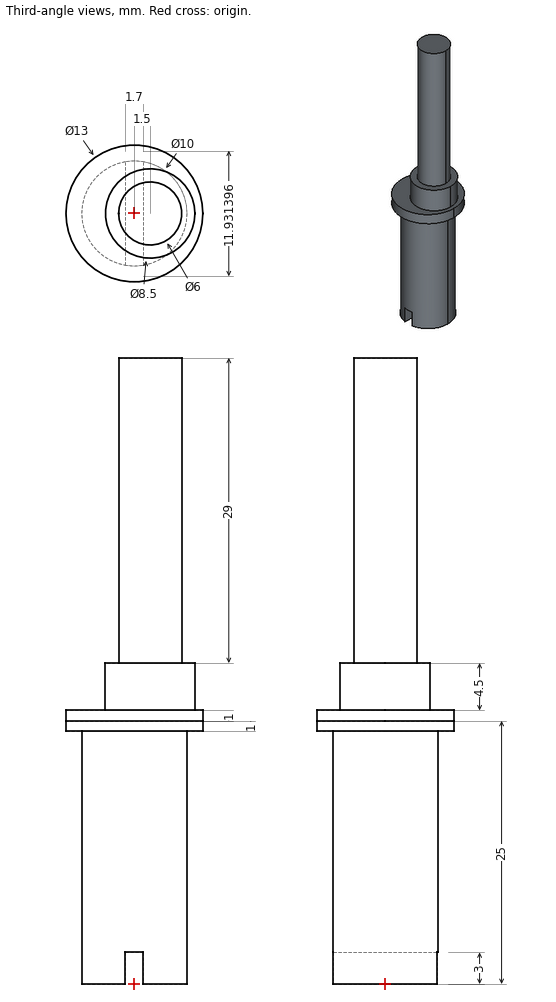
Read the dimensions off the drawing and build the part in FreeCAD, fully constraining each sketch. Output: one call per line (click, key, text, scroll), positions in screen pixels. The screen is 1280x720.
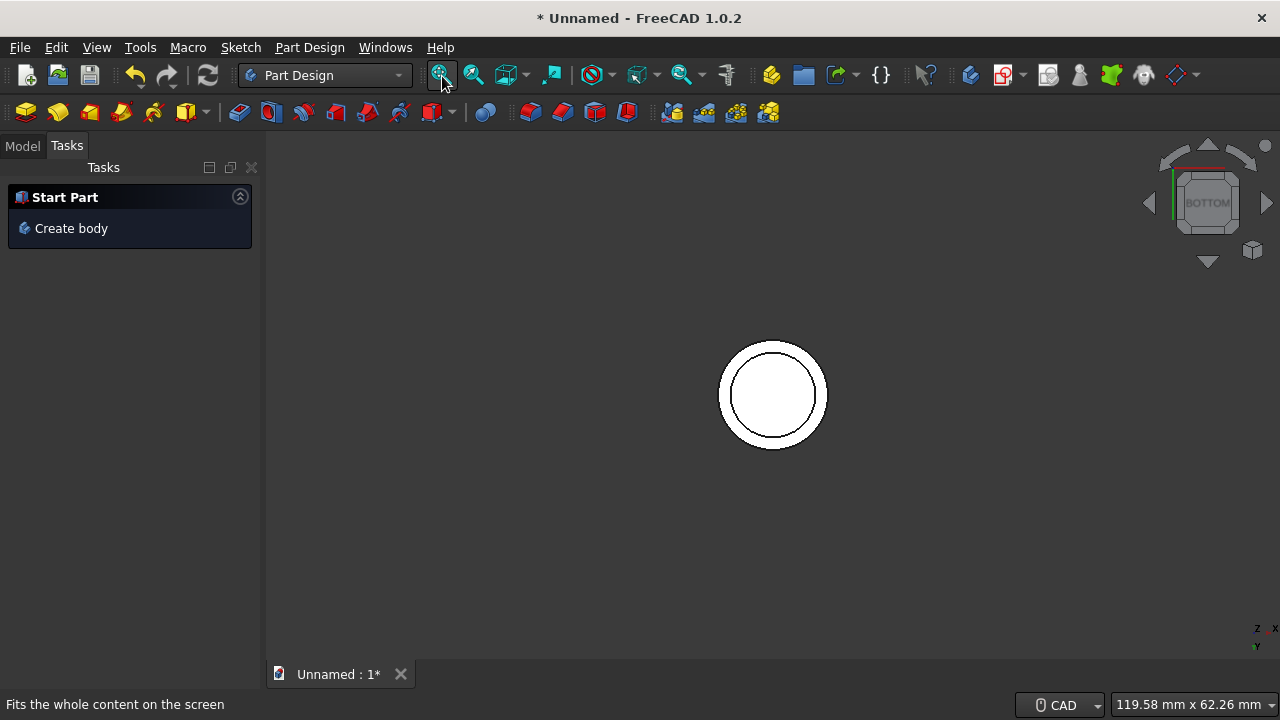
click(442, 76)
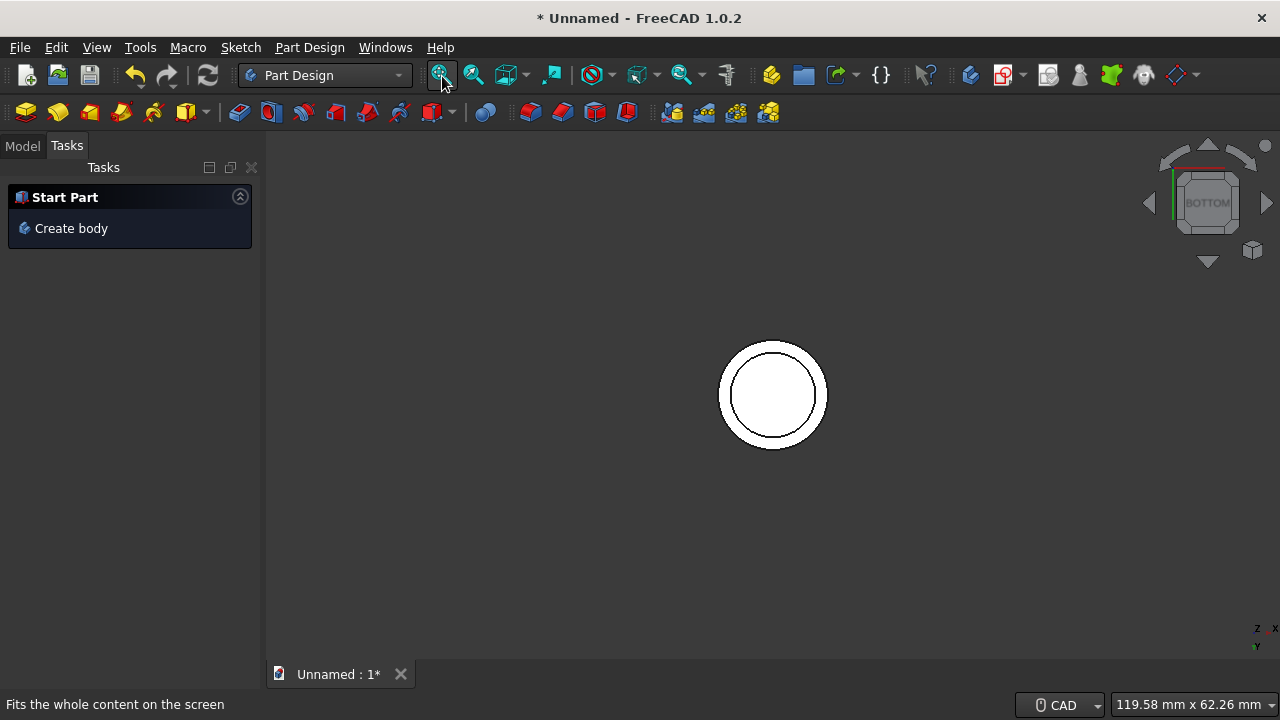
click(773, 394)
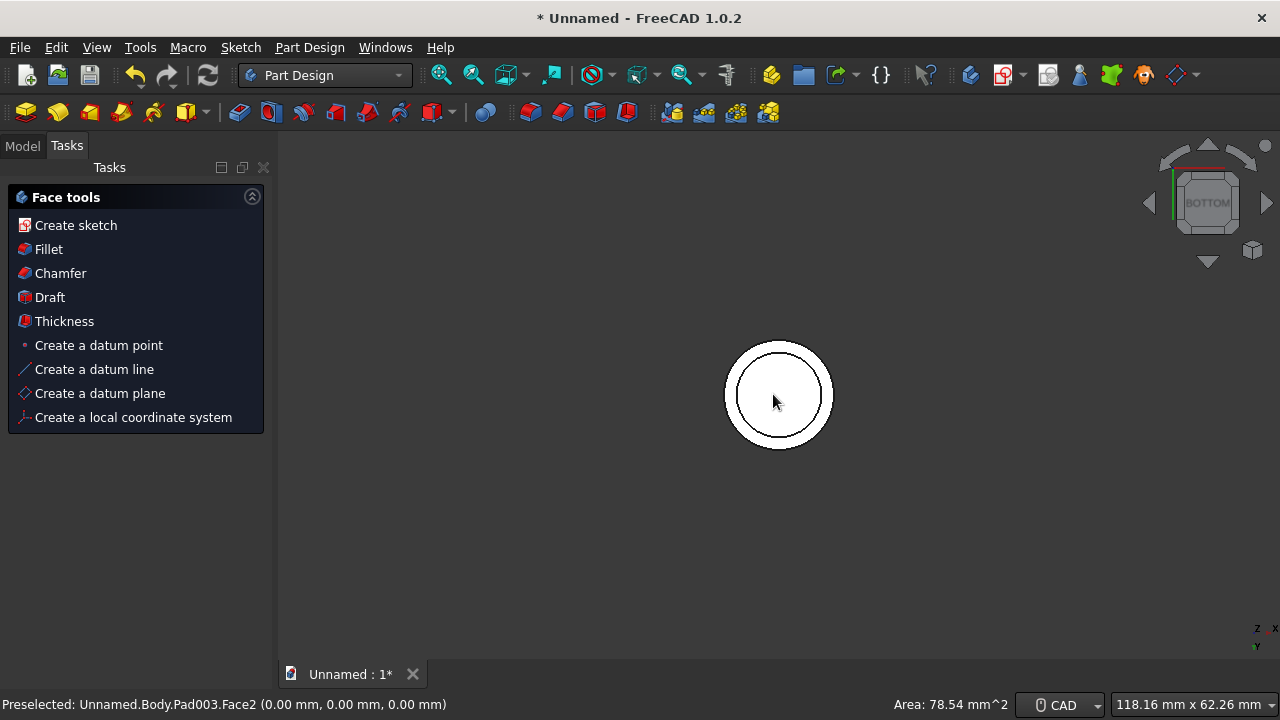
click(1004, 76)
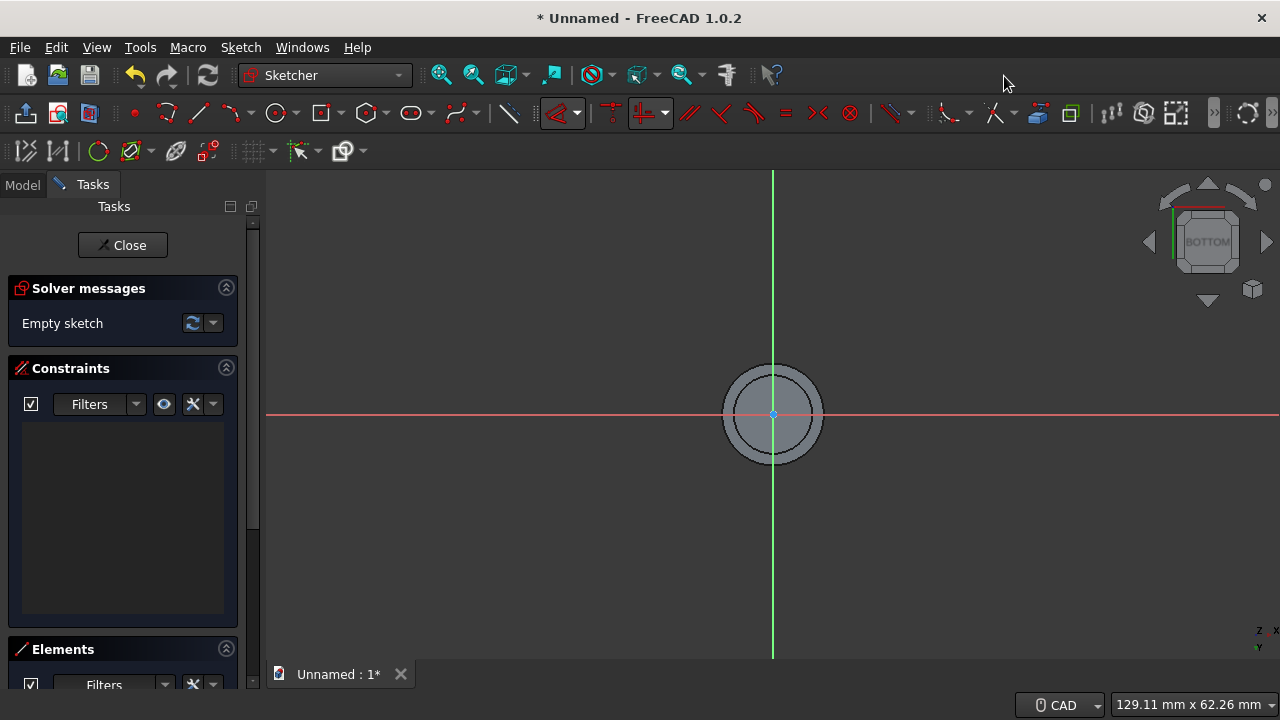
scroll(803, 415, up, 6)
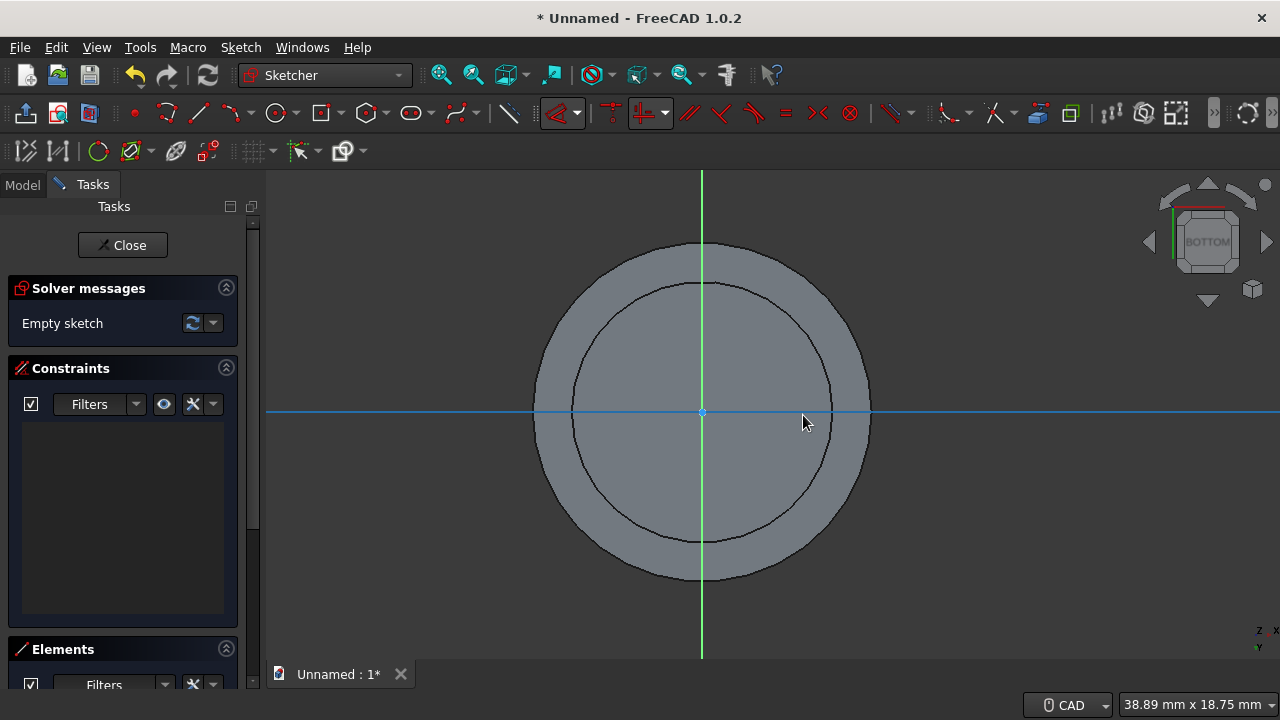
click(322, 114)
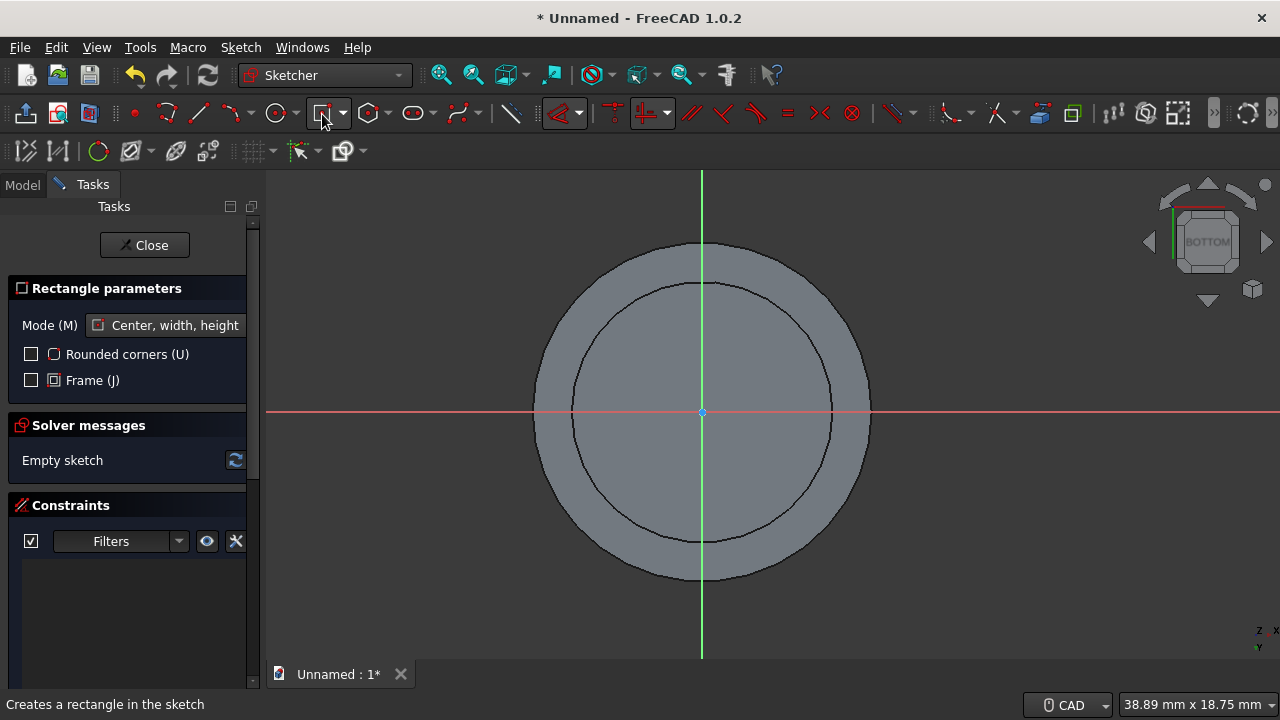
click(702, 412)
move(724, 257)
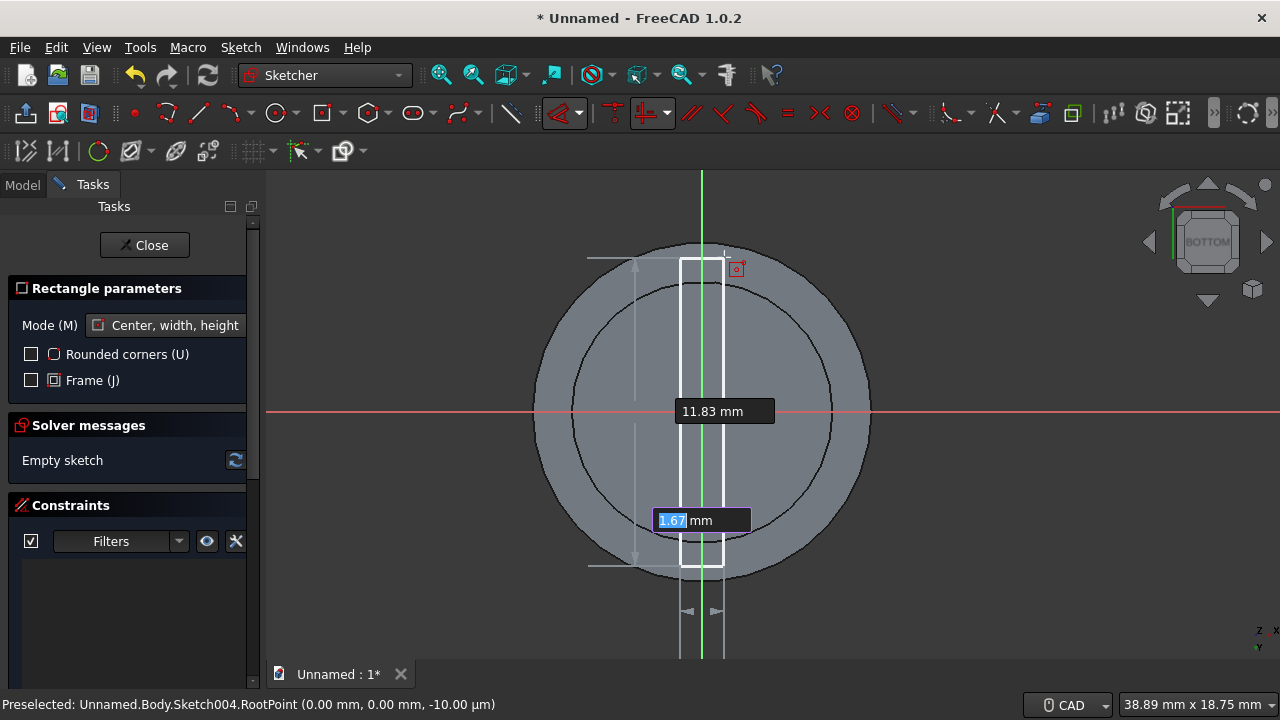
text(1.7)
key(Tab)
text(11.931396)
key(Return)
key(Escape)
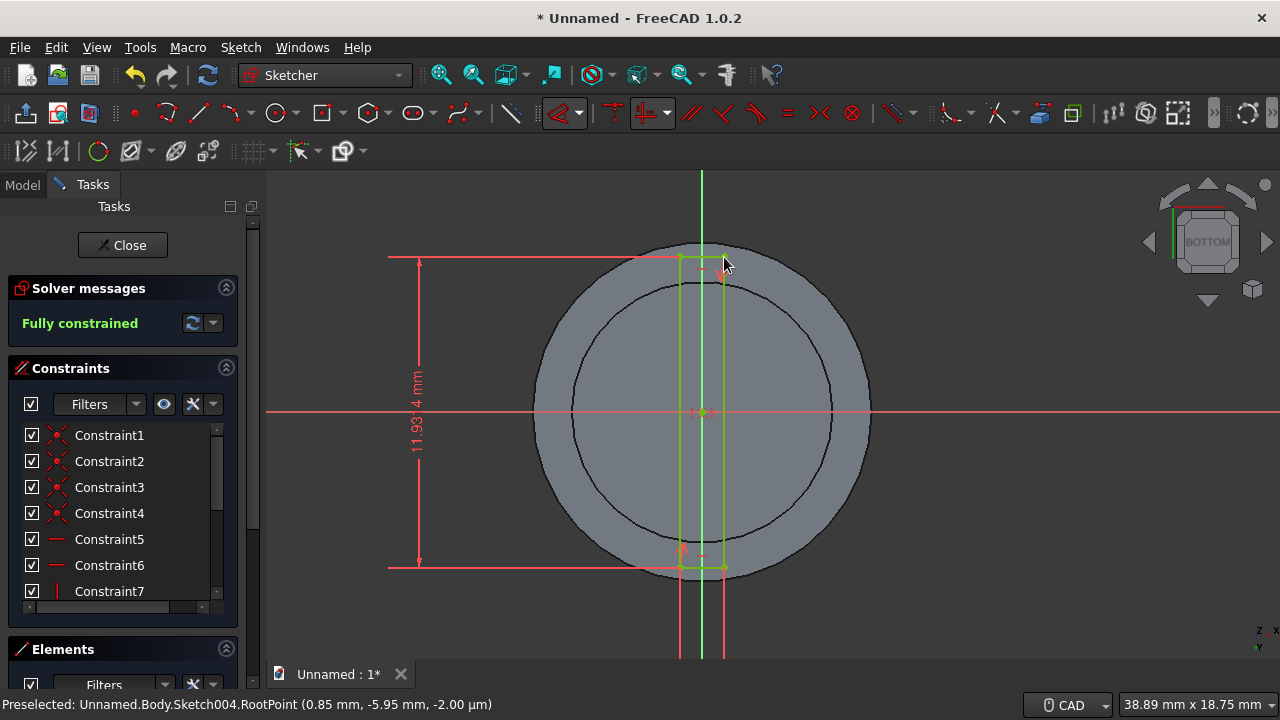
click(123, 245)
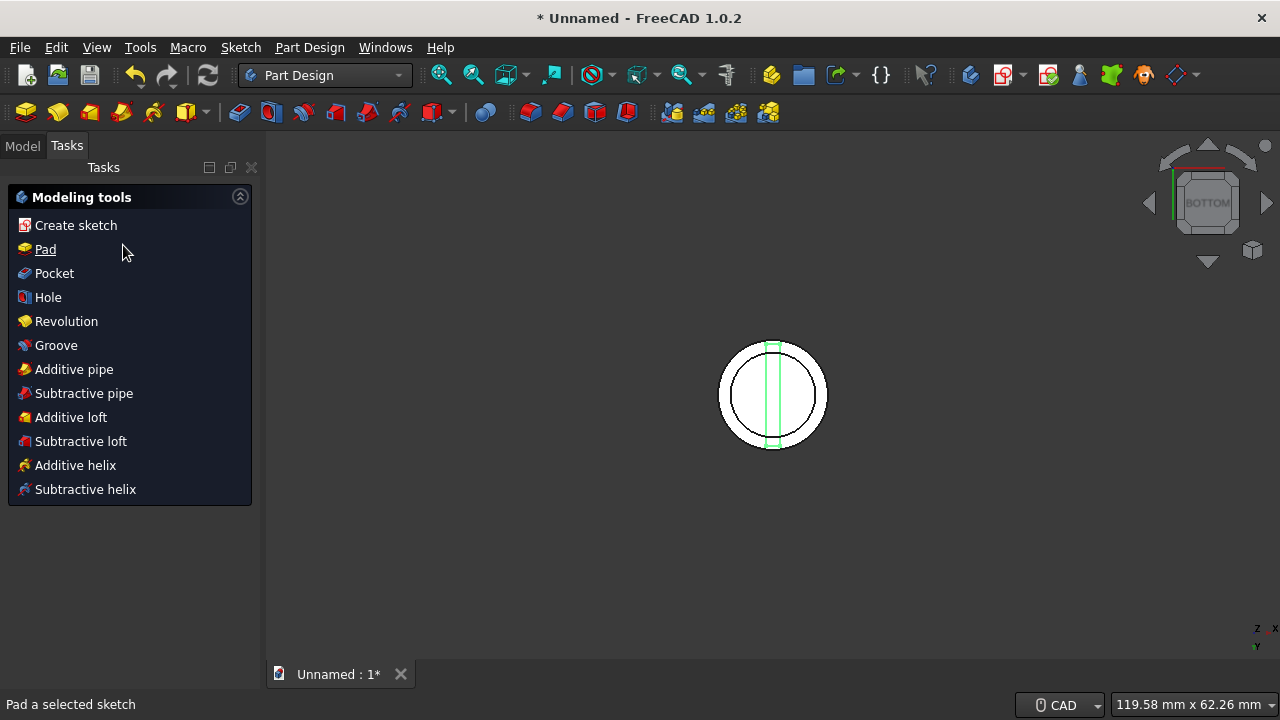
click(240, 112)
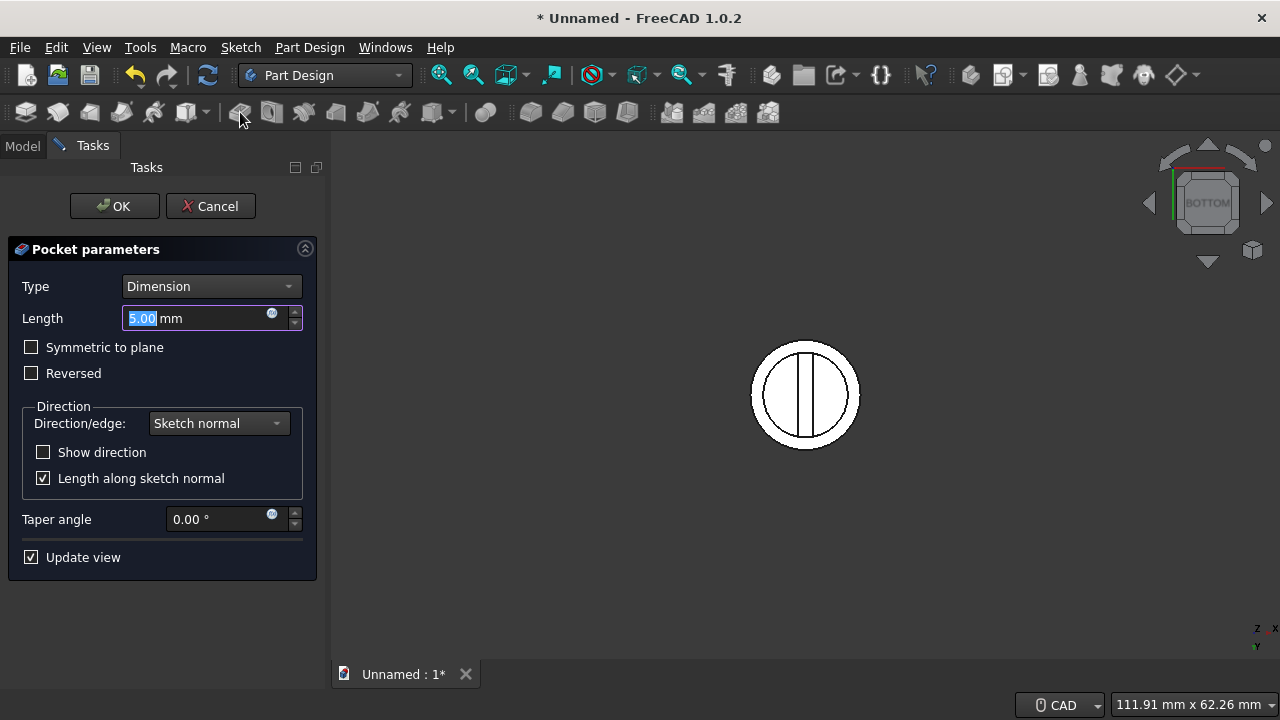
text(3)
key(Tab)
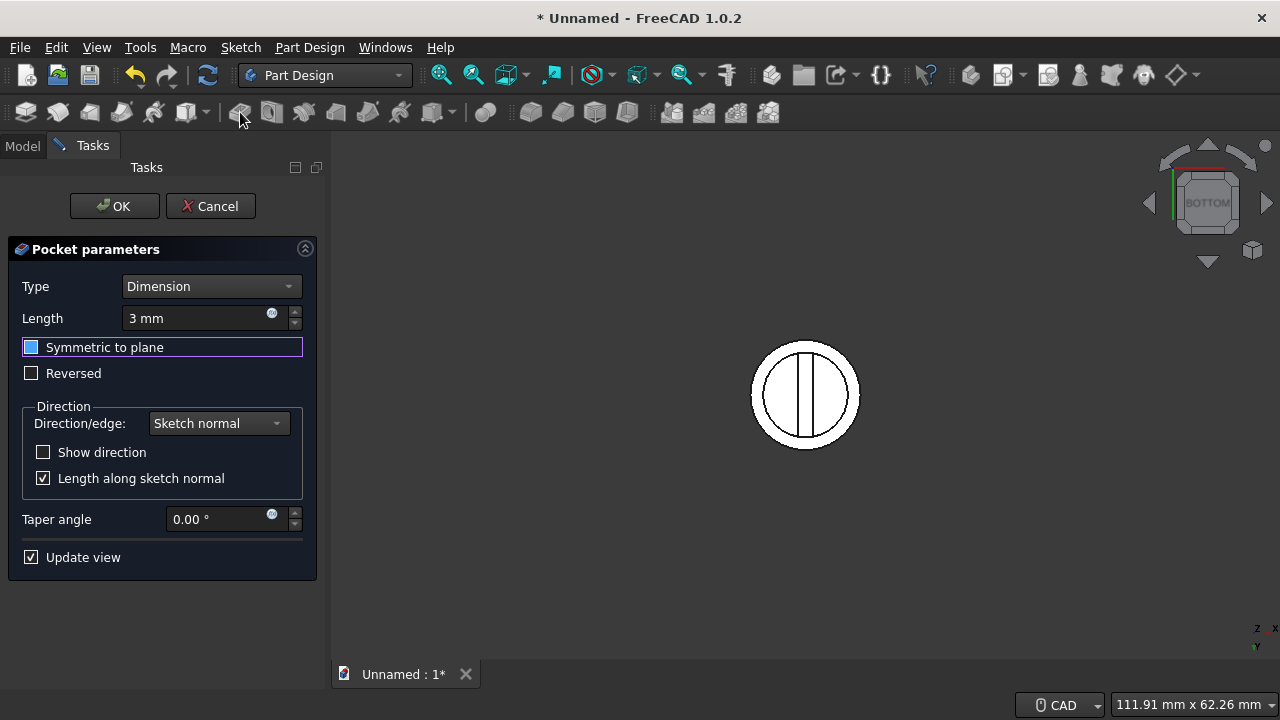
click(115, 206)